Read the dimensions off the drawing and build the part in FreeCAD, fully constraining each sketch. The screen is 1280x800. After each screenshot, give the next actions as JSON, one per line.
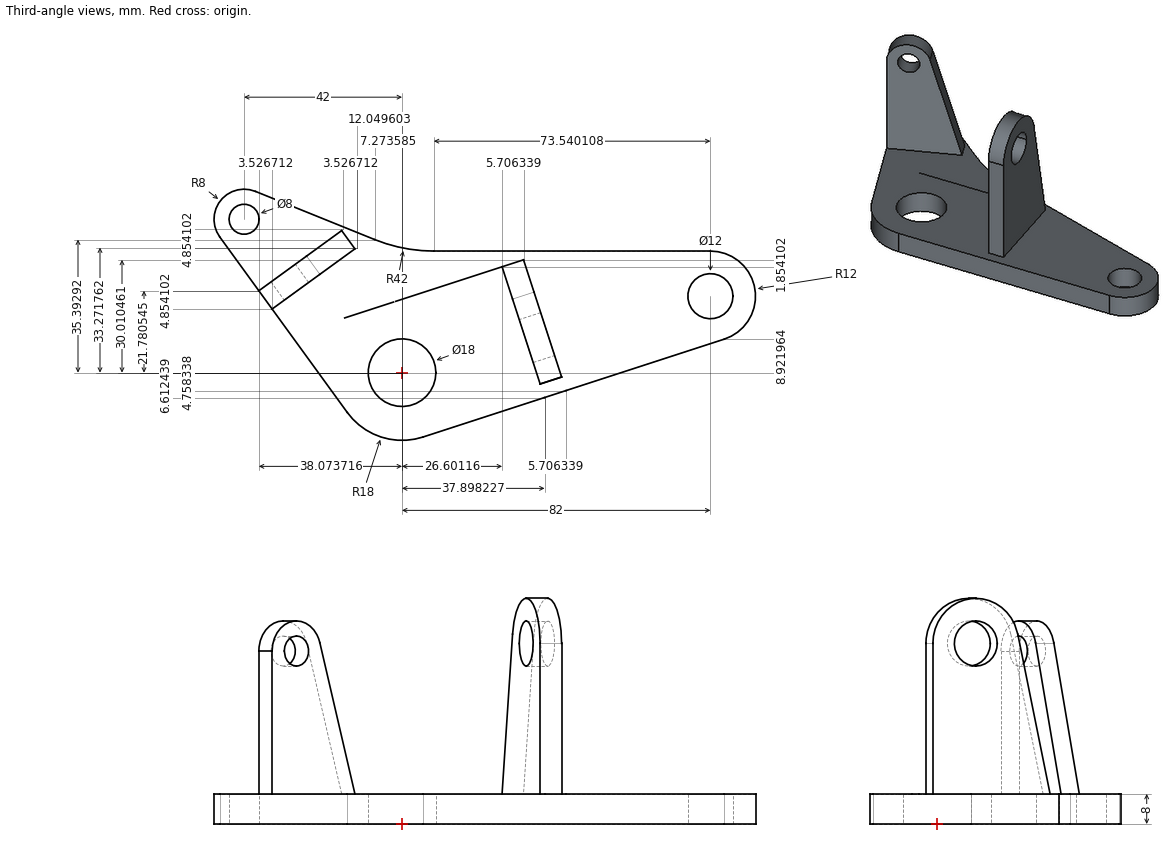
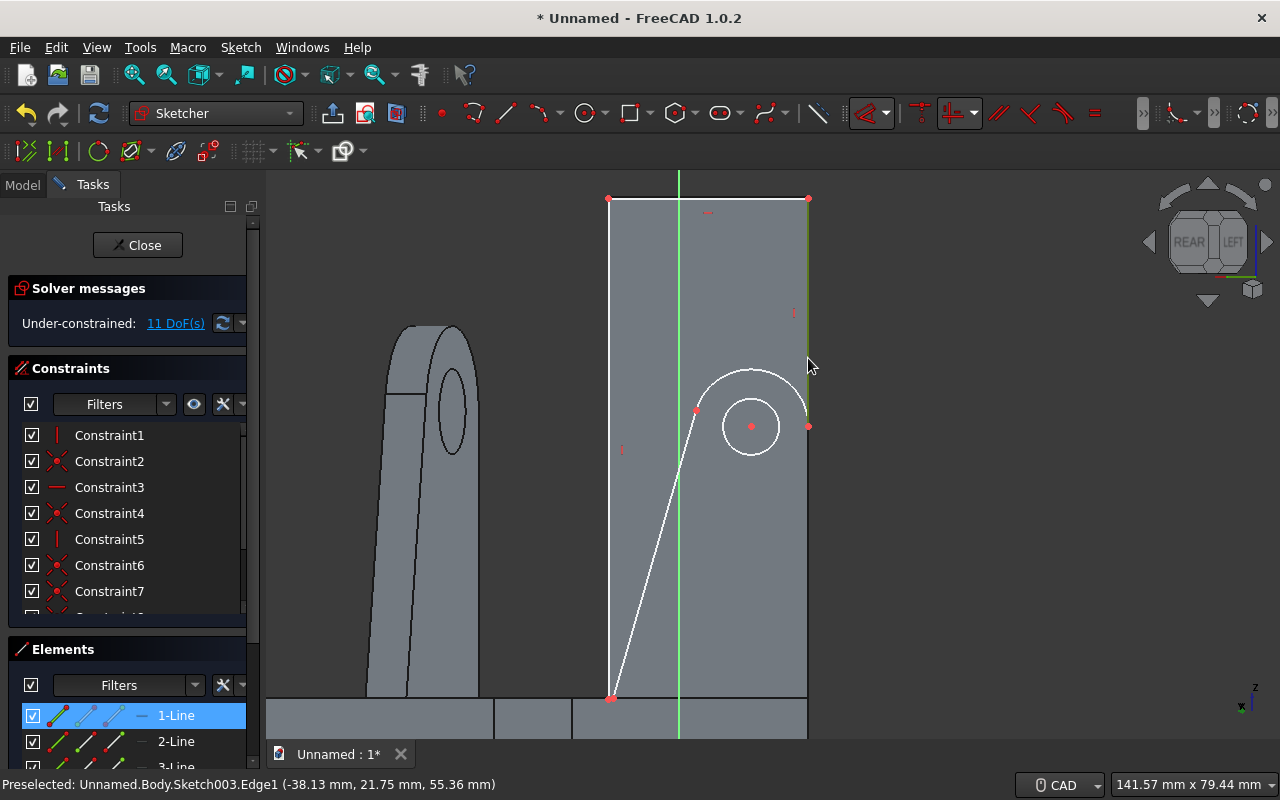
{"action": "left_click", "coordinate": [789, 383]}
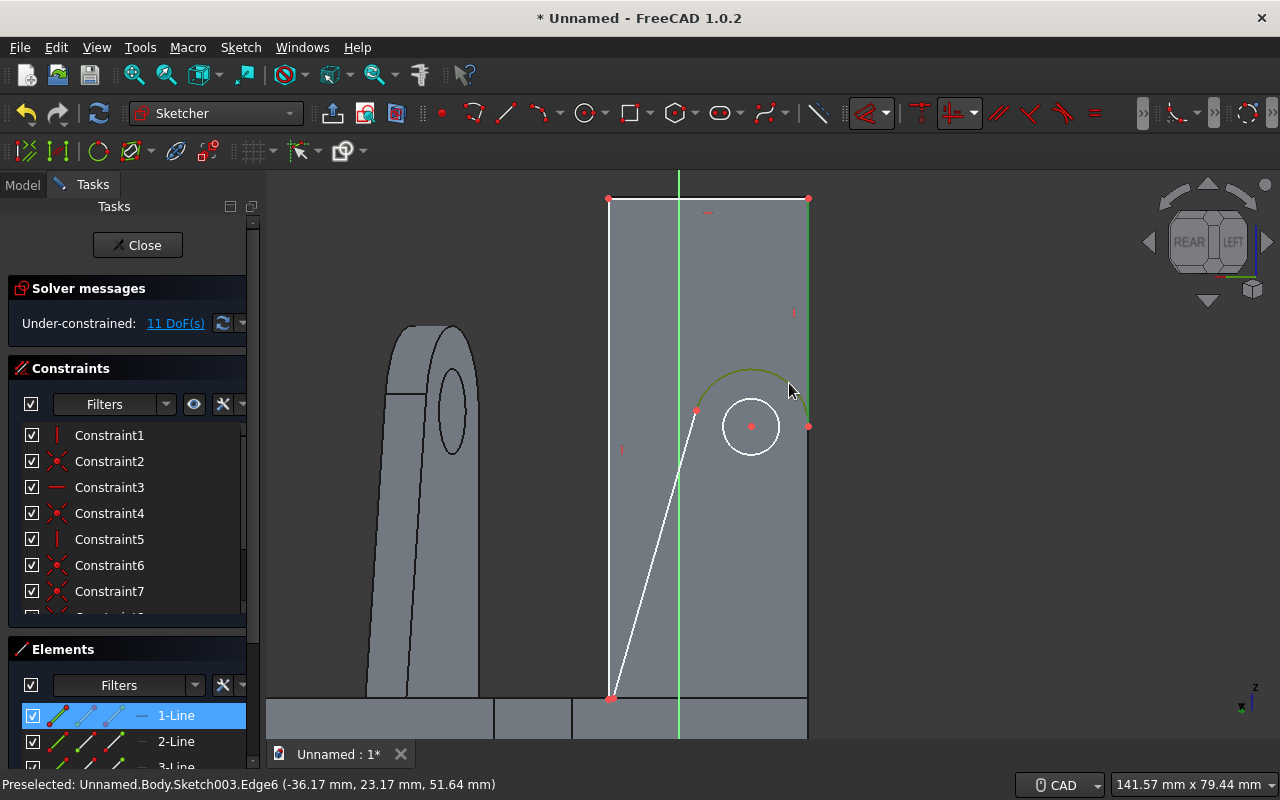
{"action": "left_click", "coordinate": [1064, 114]}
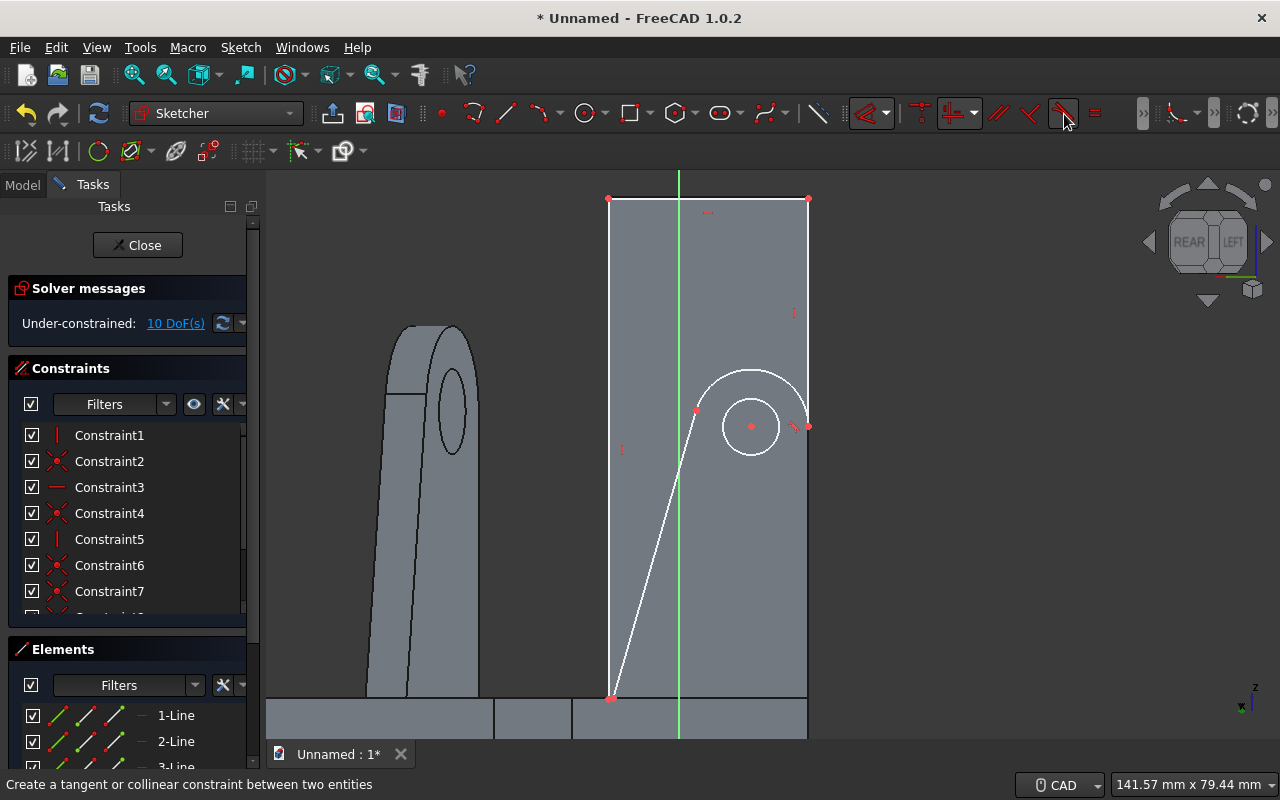
{"action": "left_click", "coordinate": [638, 612]}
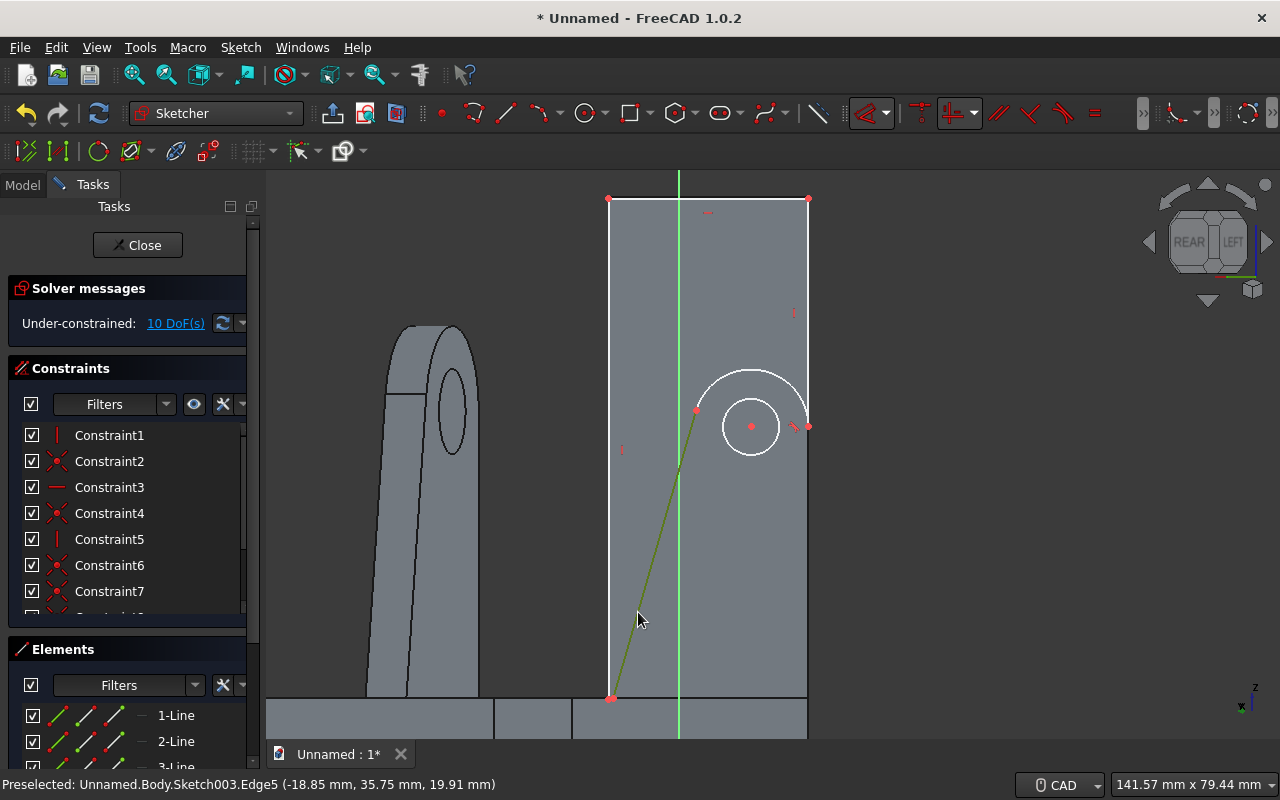
{"action": "left_click", "coordinate": [789, 384]}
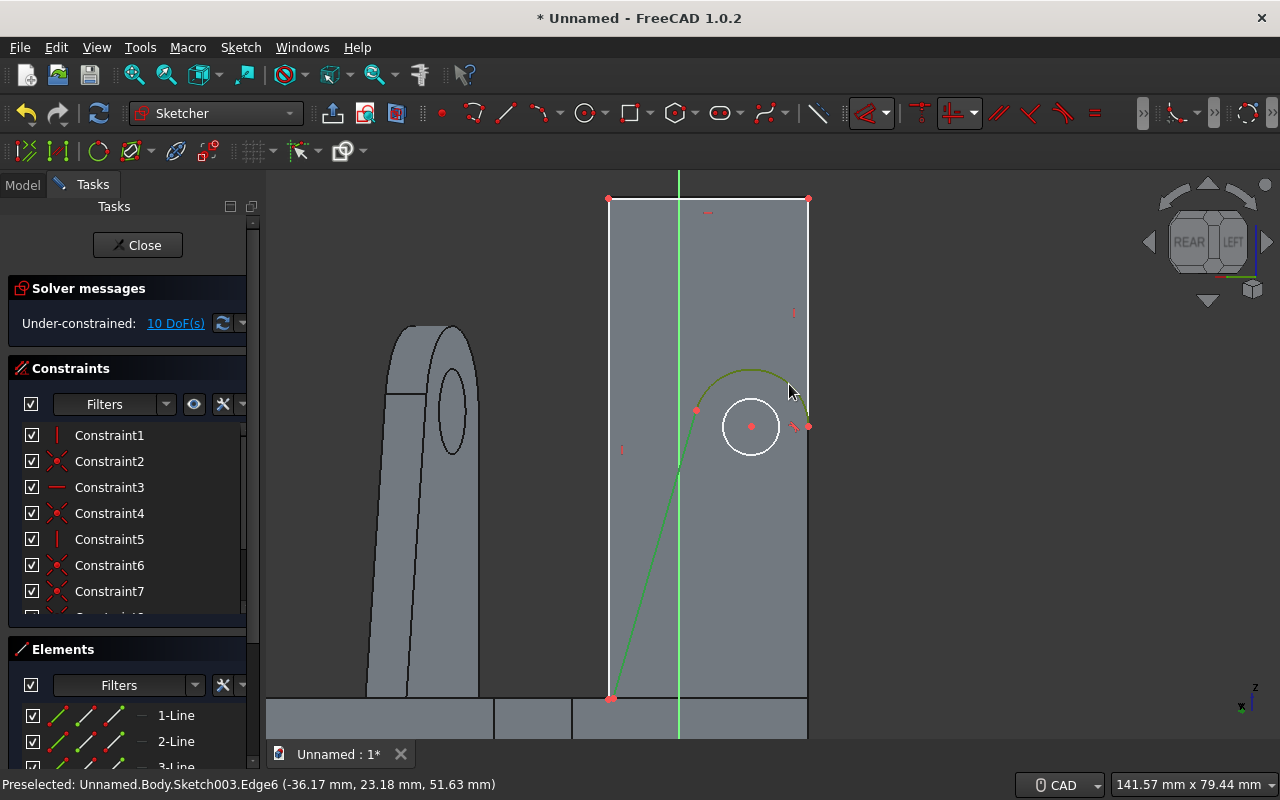
{"action": "key", "text": "t"}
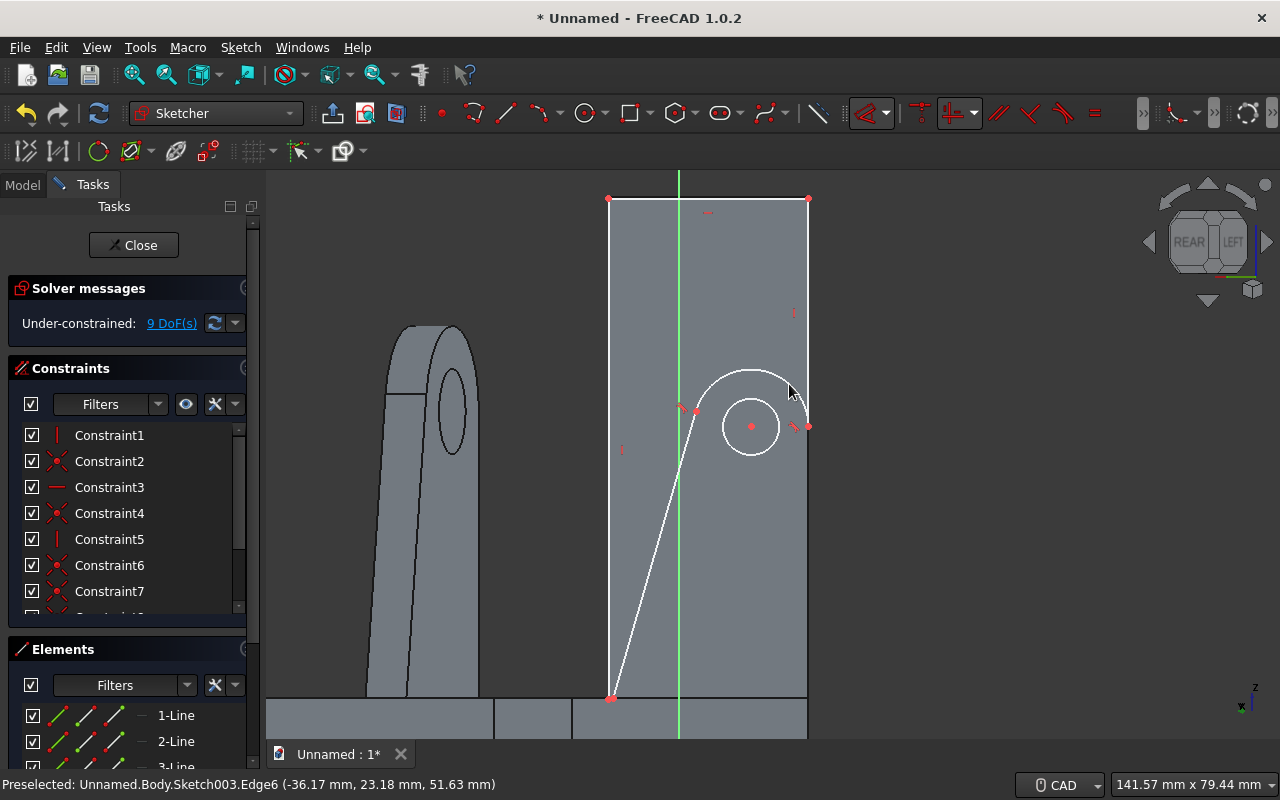
{"action": "scroll", "coordinate": [611, 699], "scroll_direction": "up", "scroll_amount": 10}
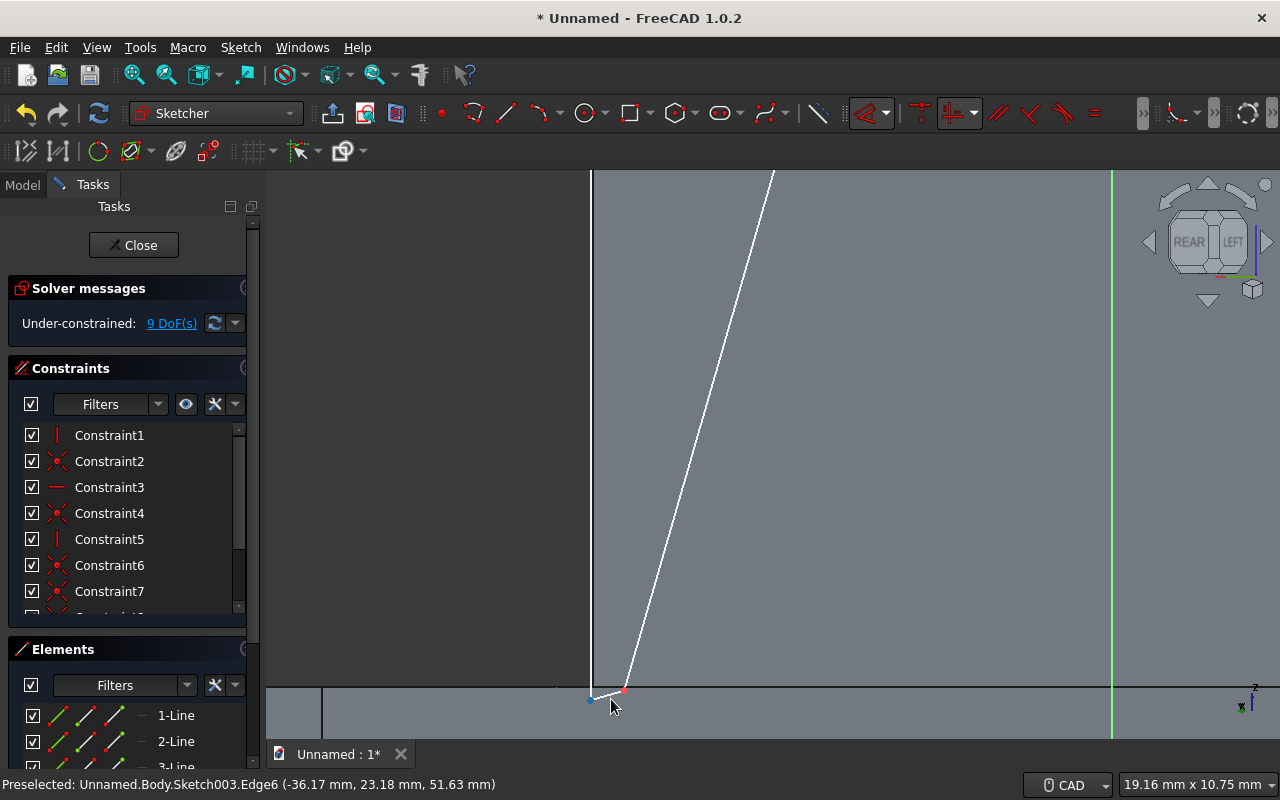
{"action": "left_click", "coordinate": [608, 695]}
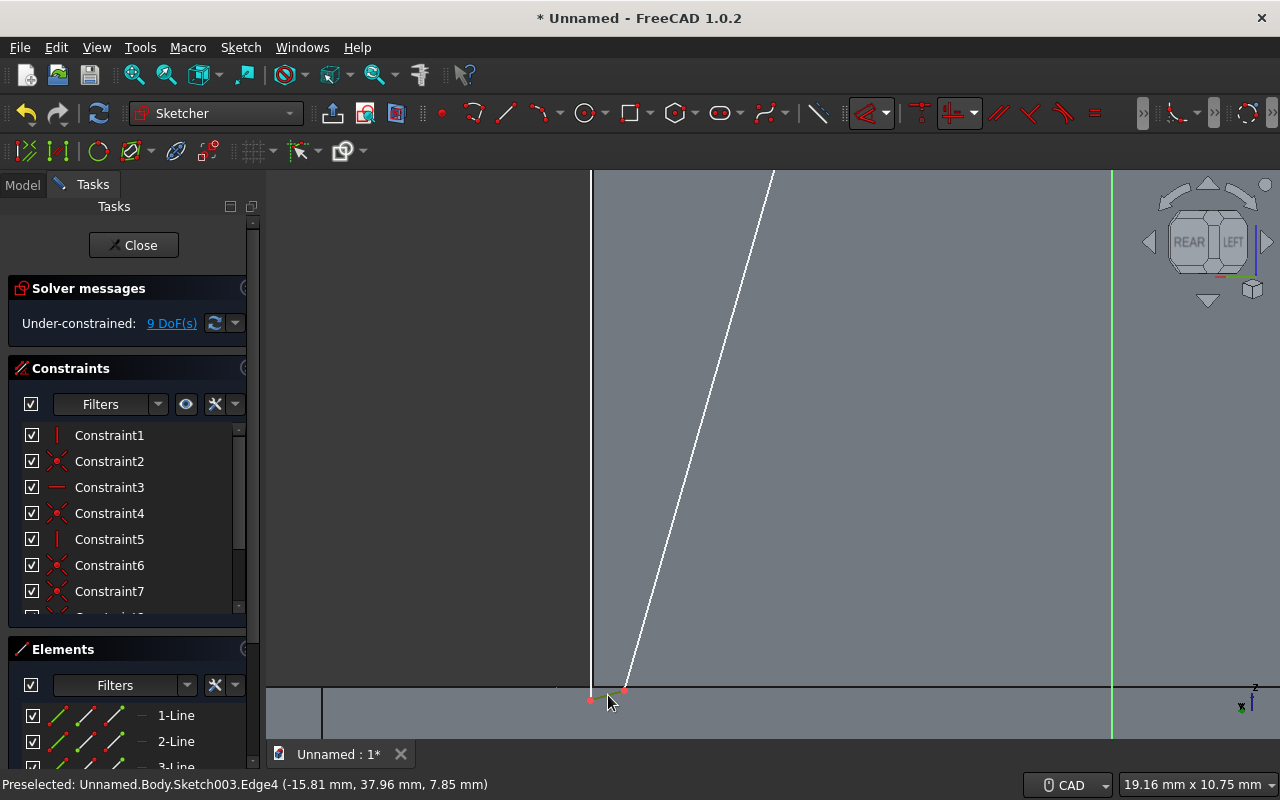
{"action": "left_click", "coordinate": [976, 114]}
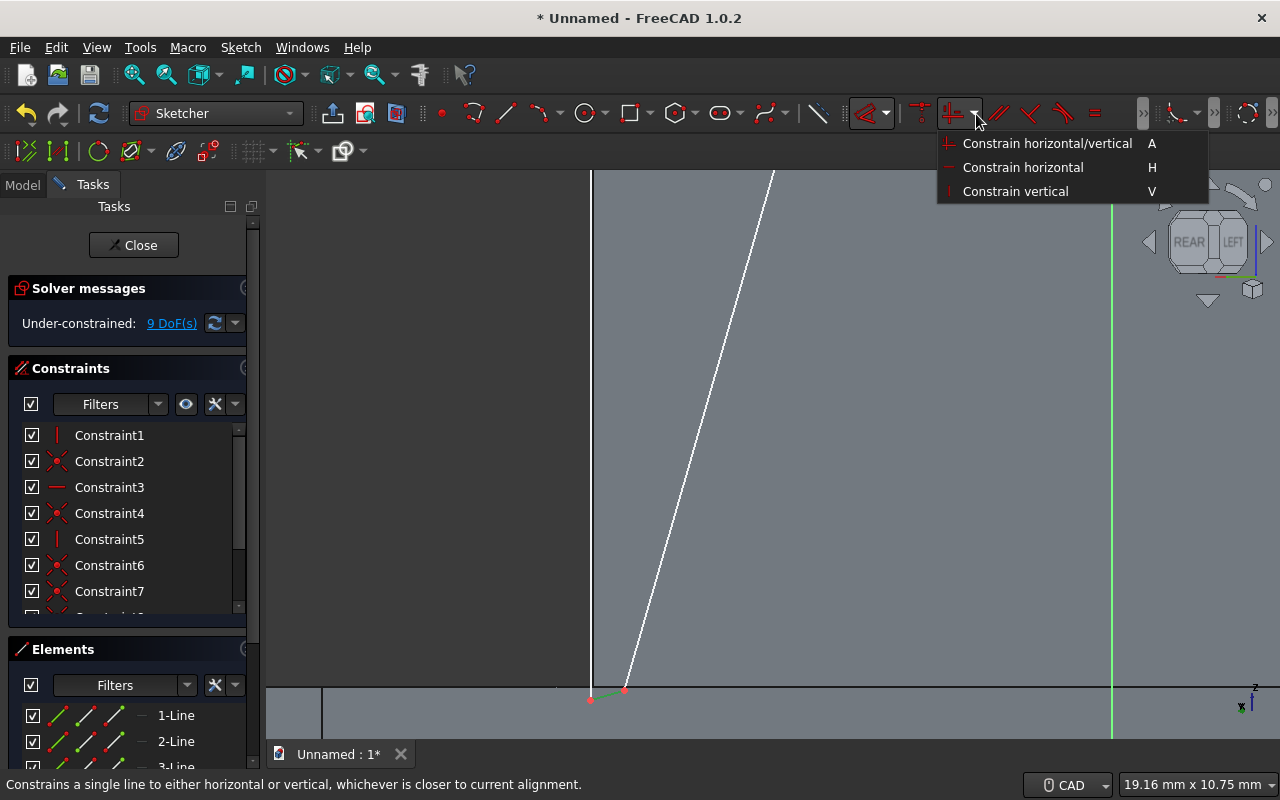
{"action": "left_click", "coordinate": [1073, 167]}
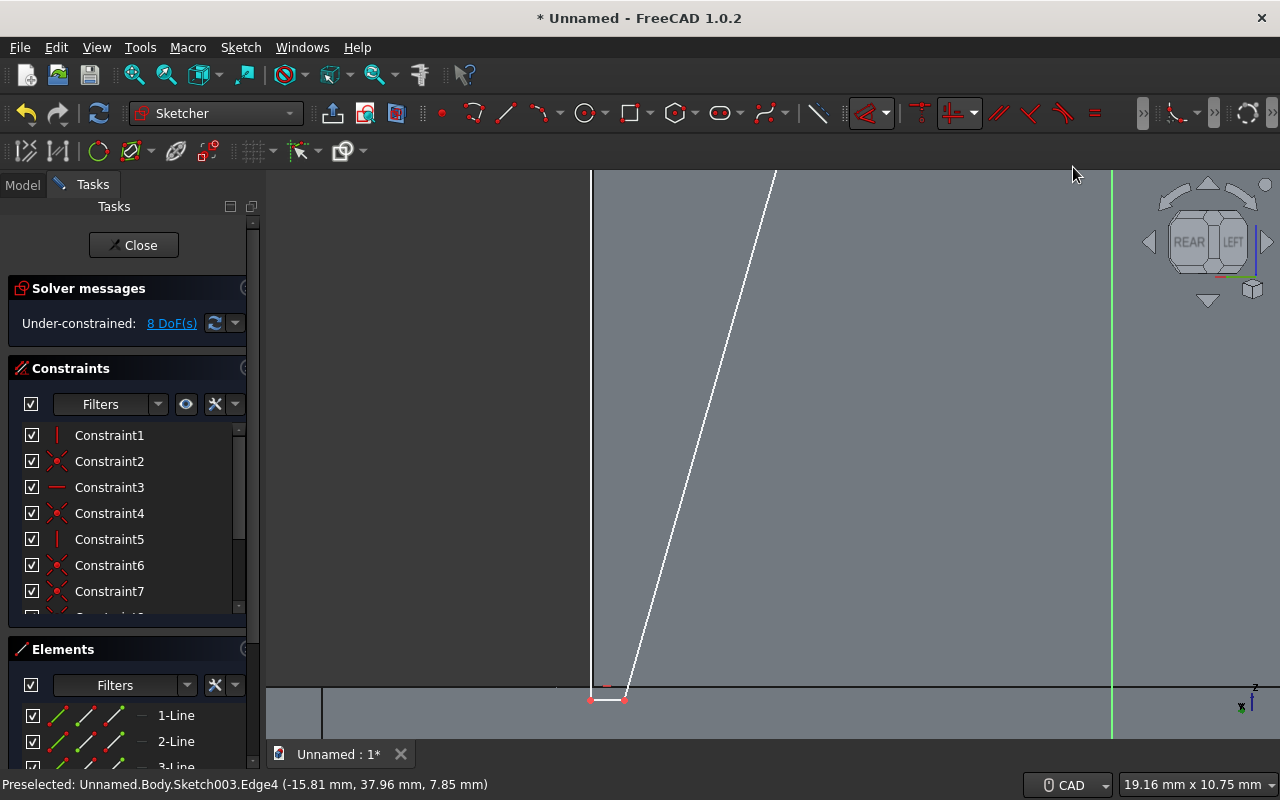
{"action": "scroll", "coordinate": [642, 595], "scroll_direction": "down", "scroll_amount": 12}